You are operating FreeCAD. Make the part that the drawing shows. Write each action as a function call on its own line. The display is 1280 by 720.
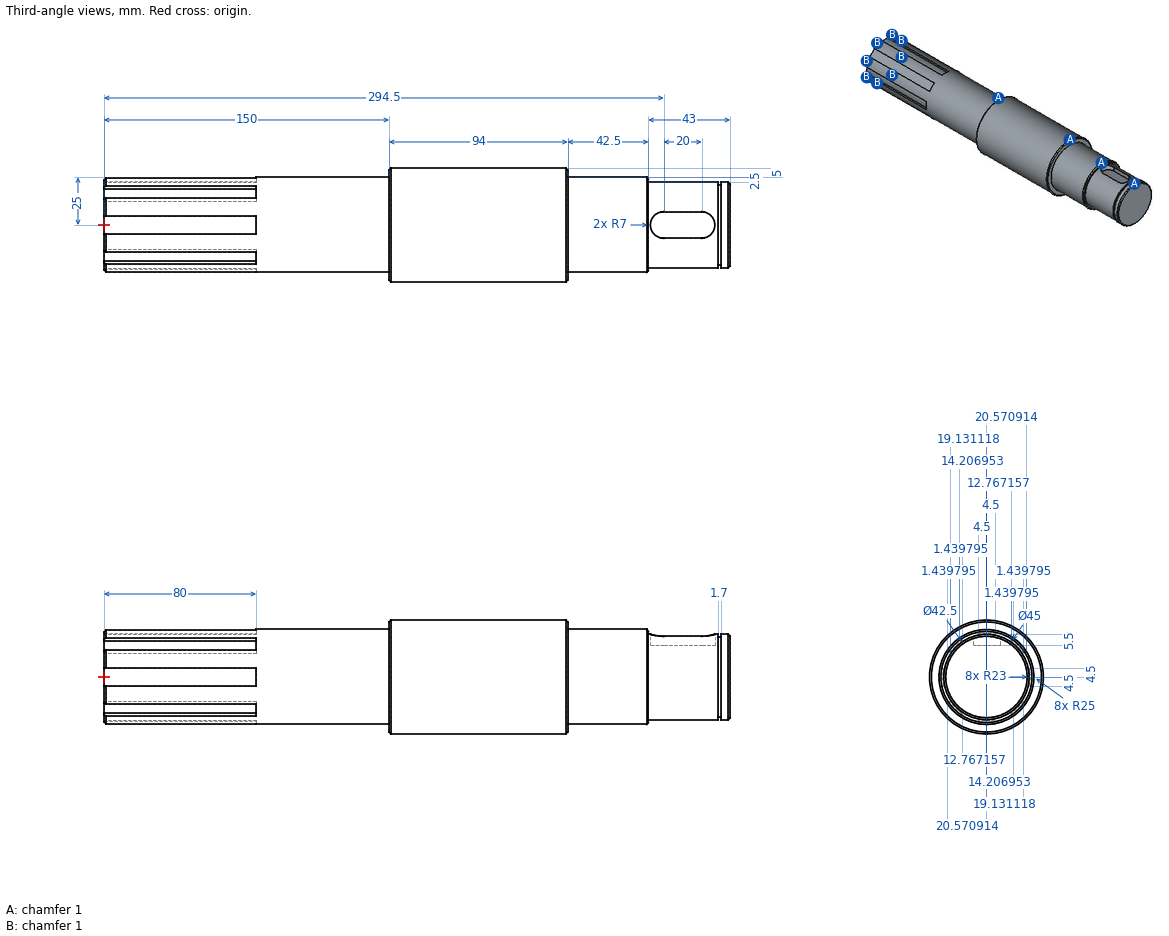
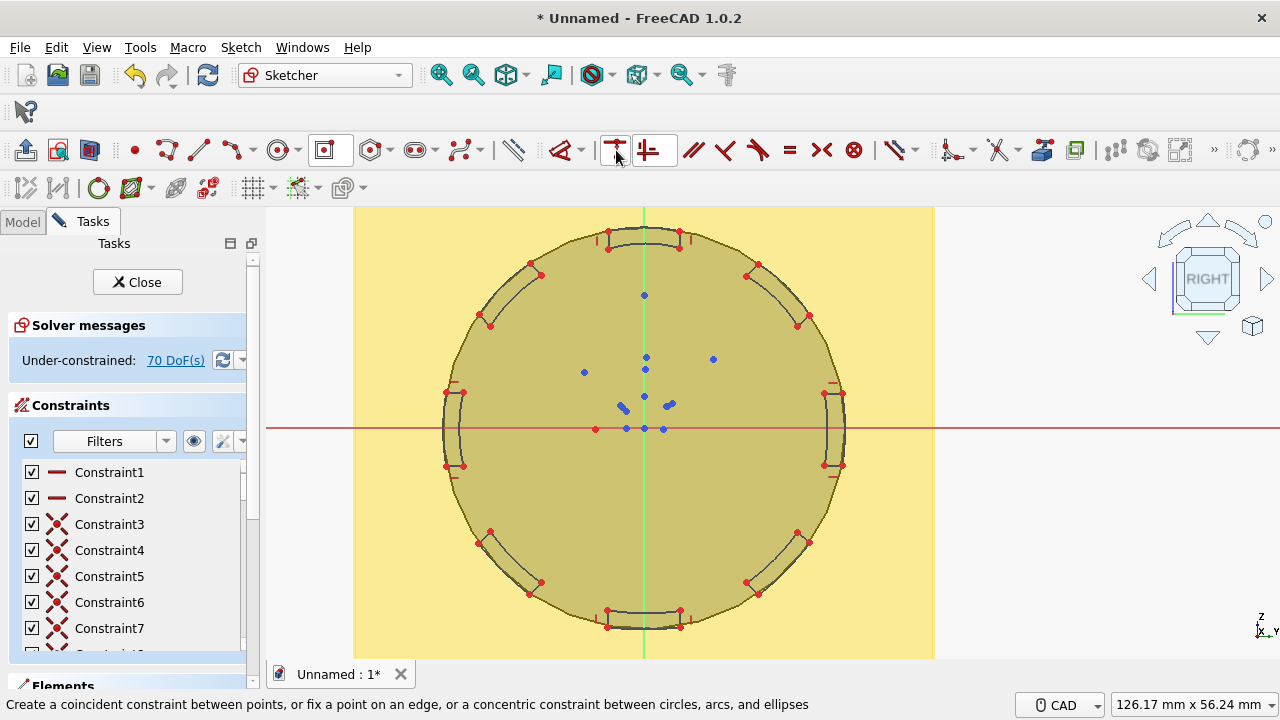
click(827, 444)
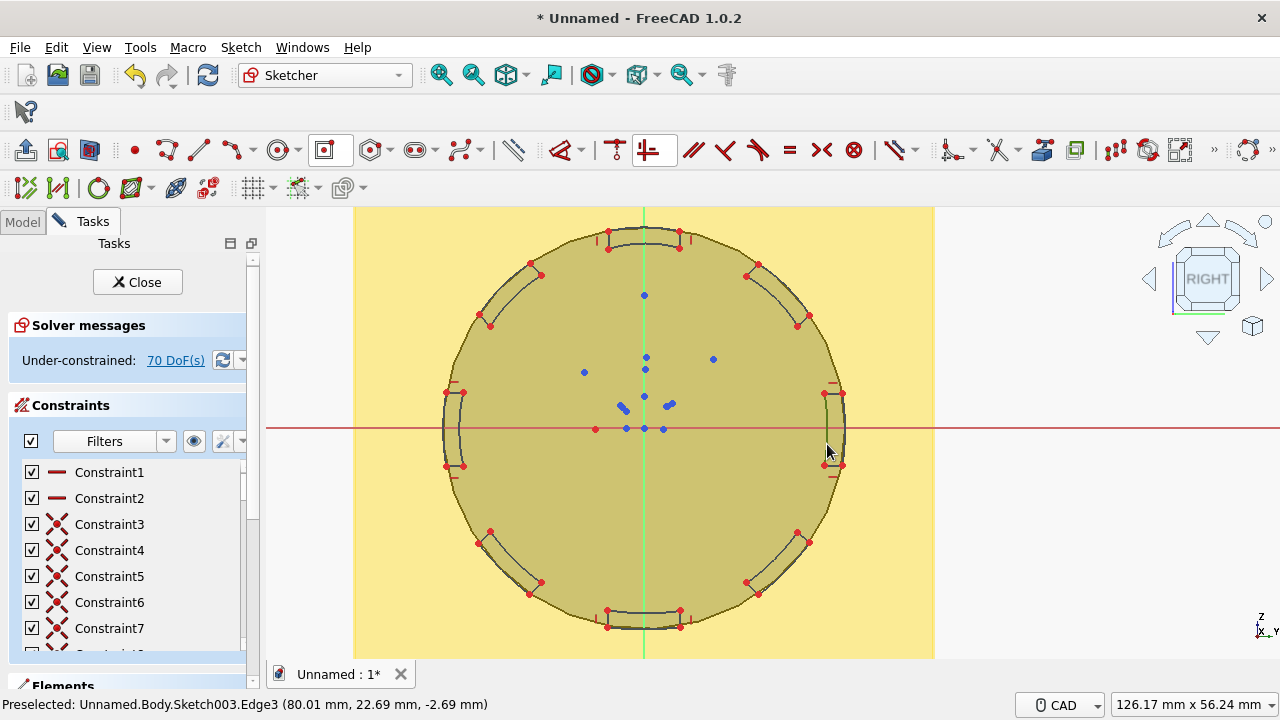
click(797, 298)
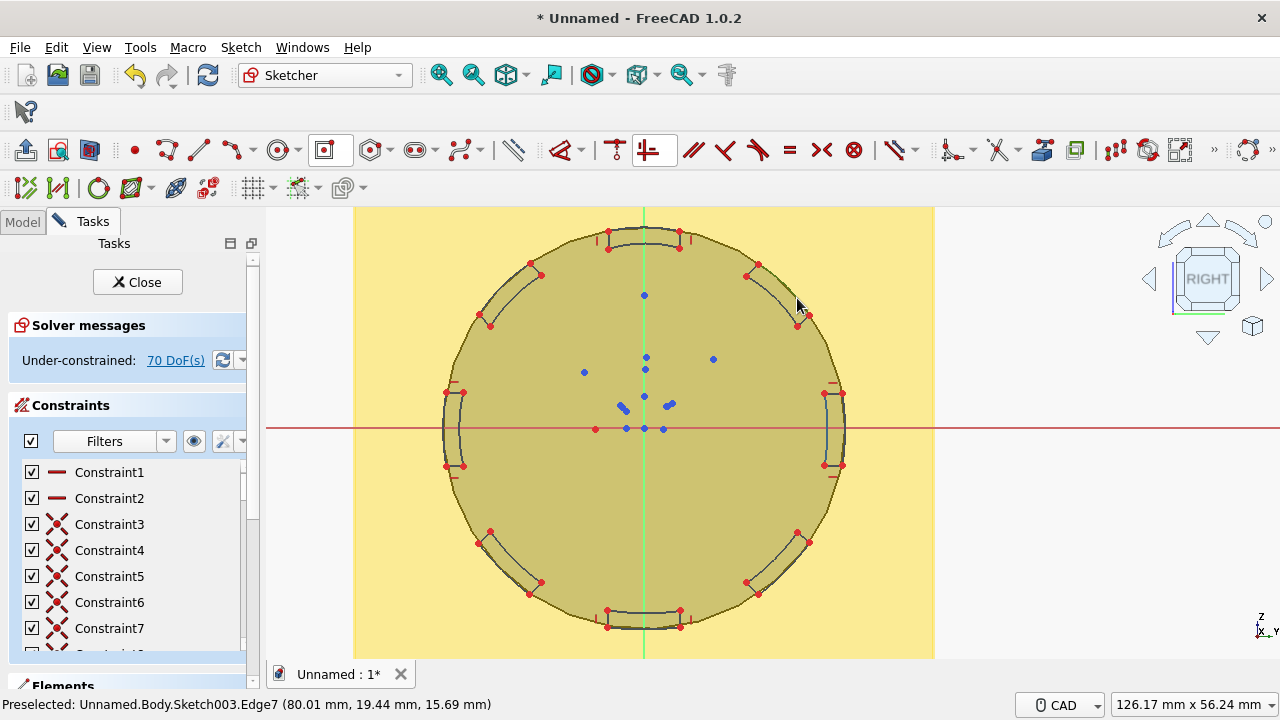
click(616, 150)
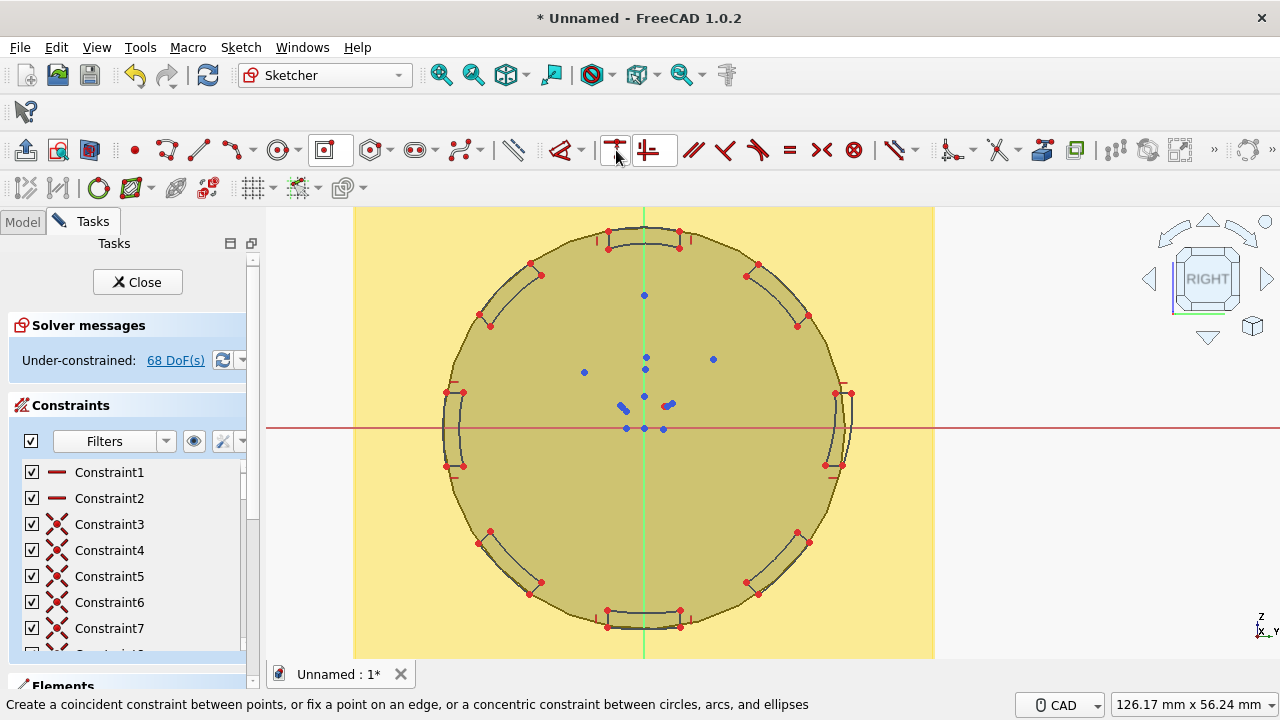
click(831, 445)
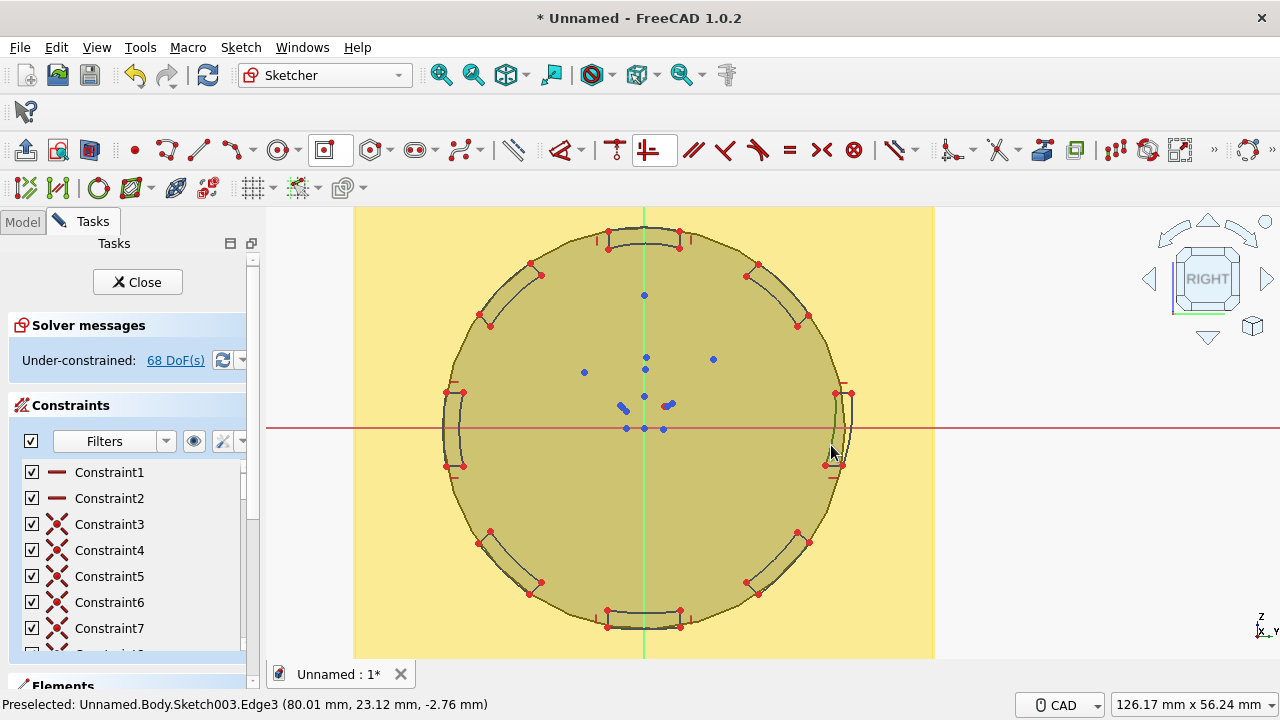
click(785, 309)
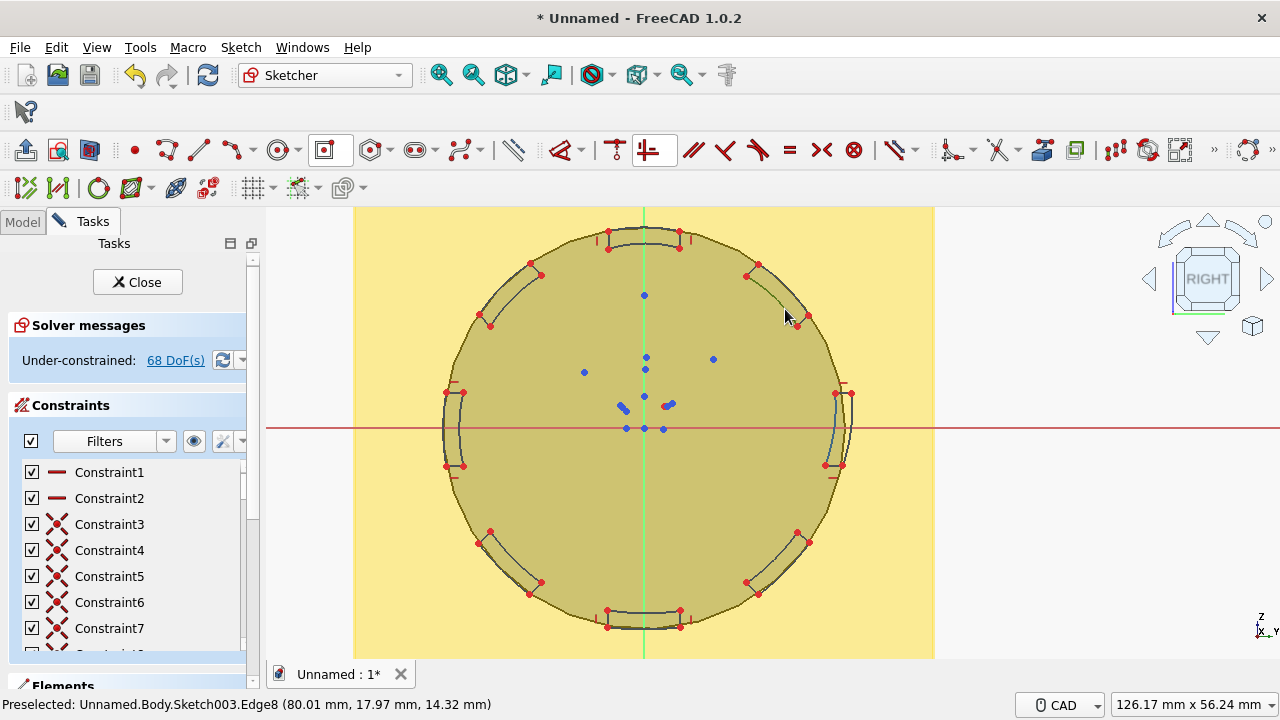
click(616, 150)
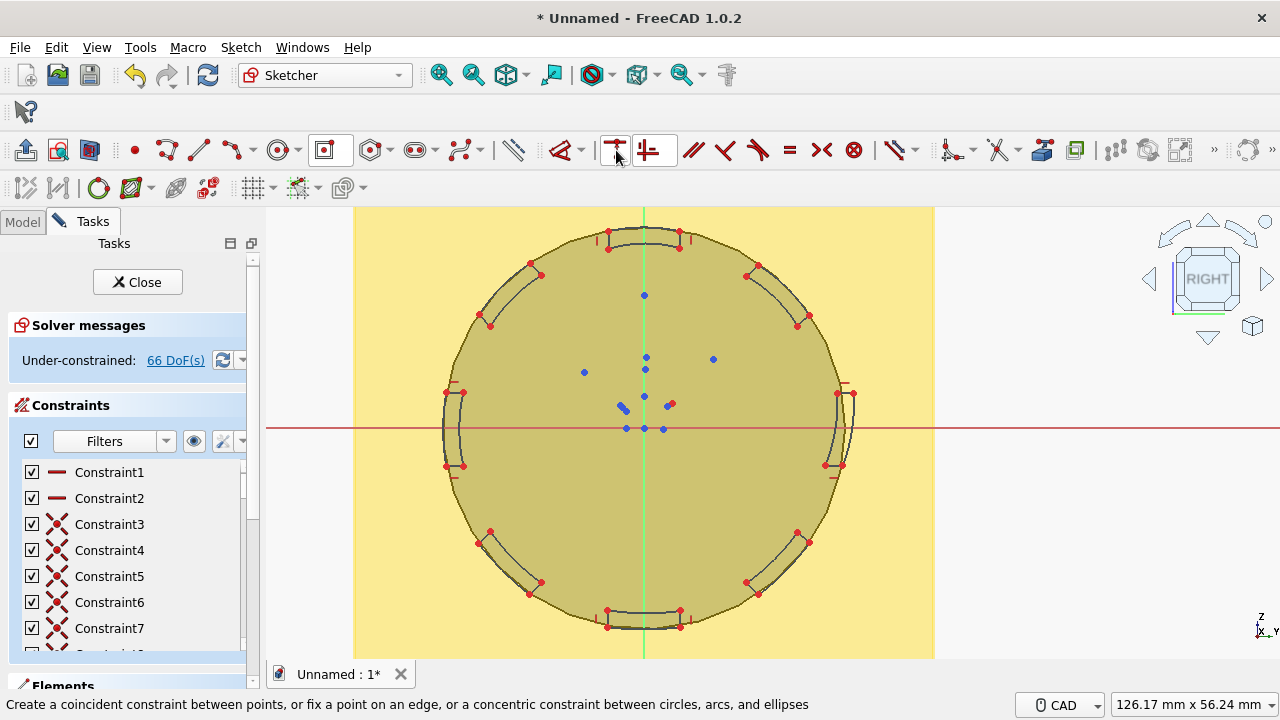
click(832, 445)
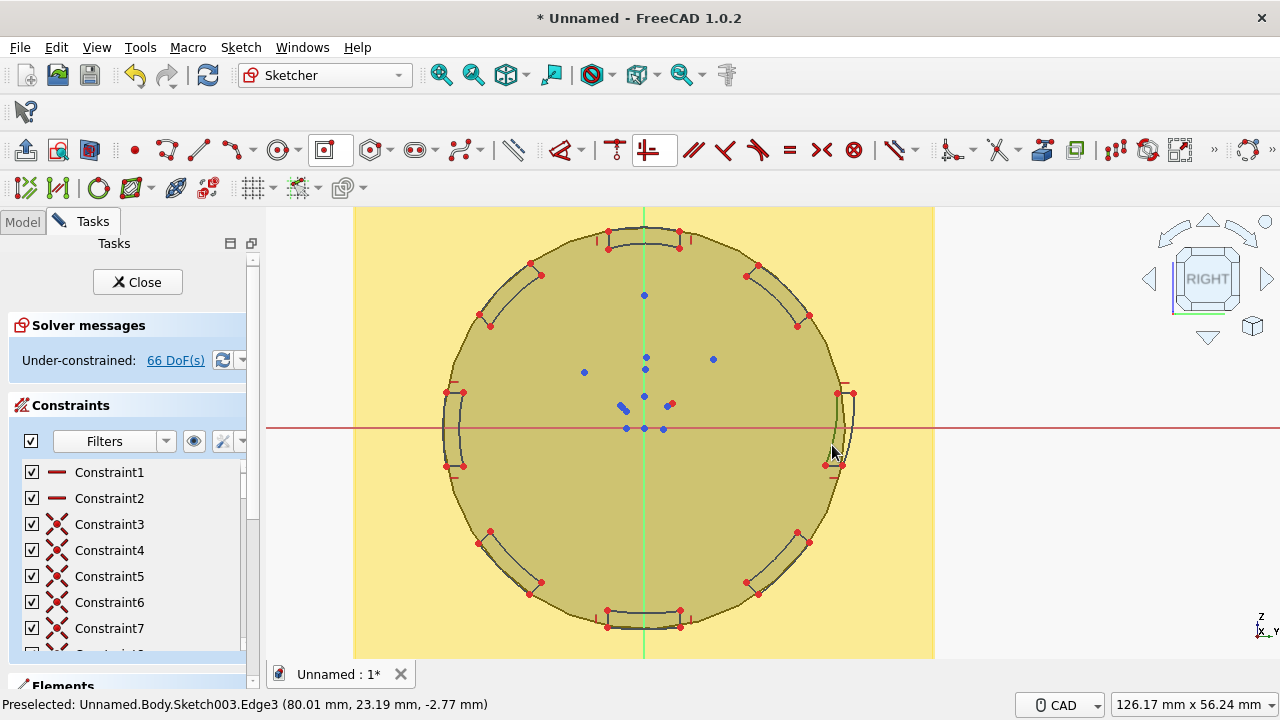
scroll(827, 443, down, 2)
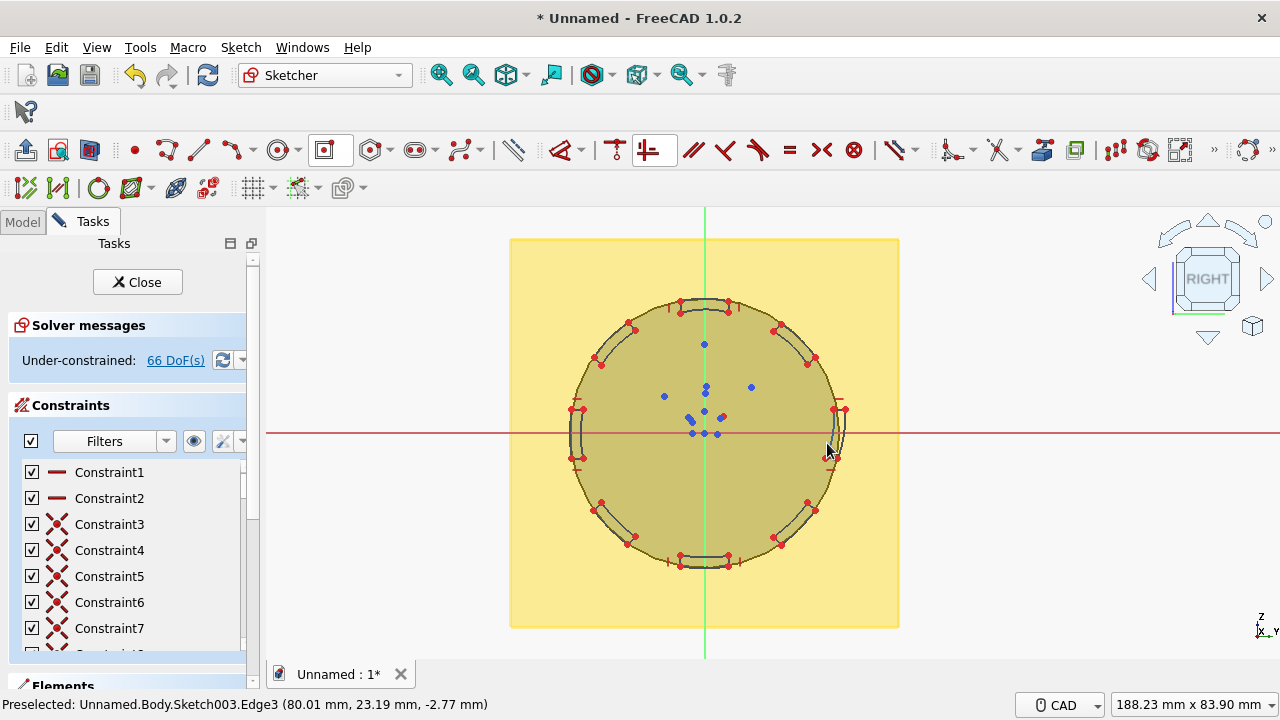
scroll(714, 299, up, 2)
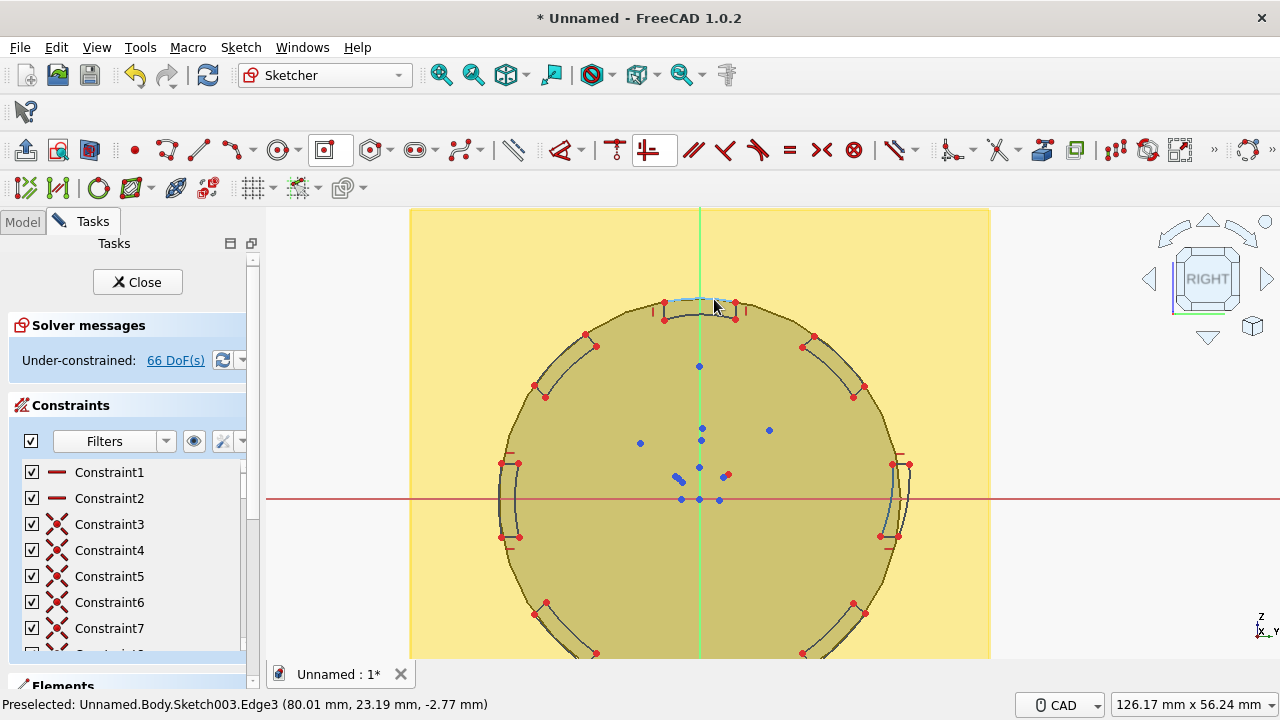
click(714, 299)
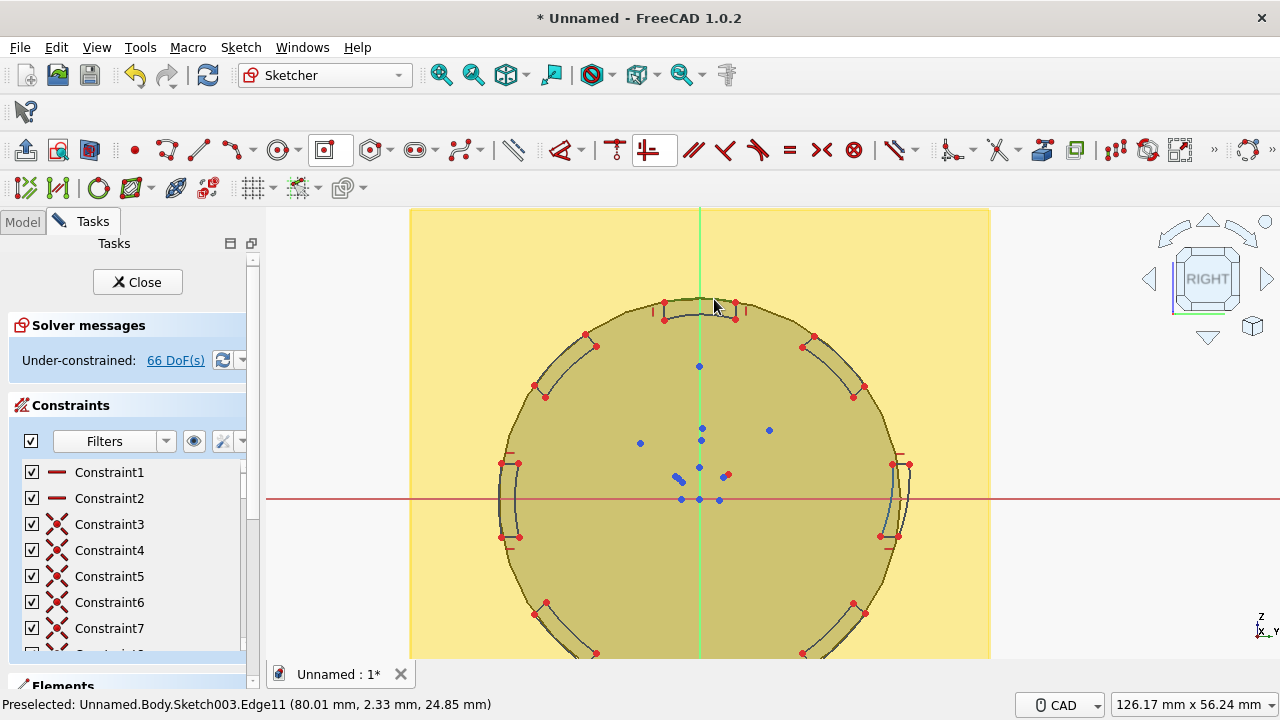
click(616, 150)